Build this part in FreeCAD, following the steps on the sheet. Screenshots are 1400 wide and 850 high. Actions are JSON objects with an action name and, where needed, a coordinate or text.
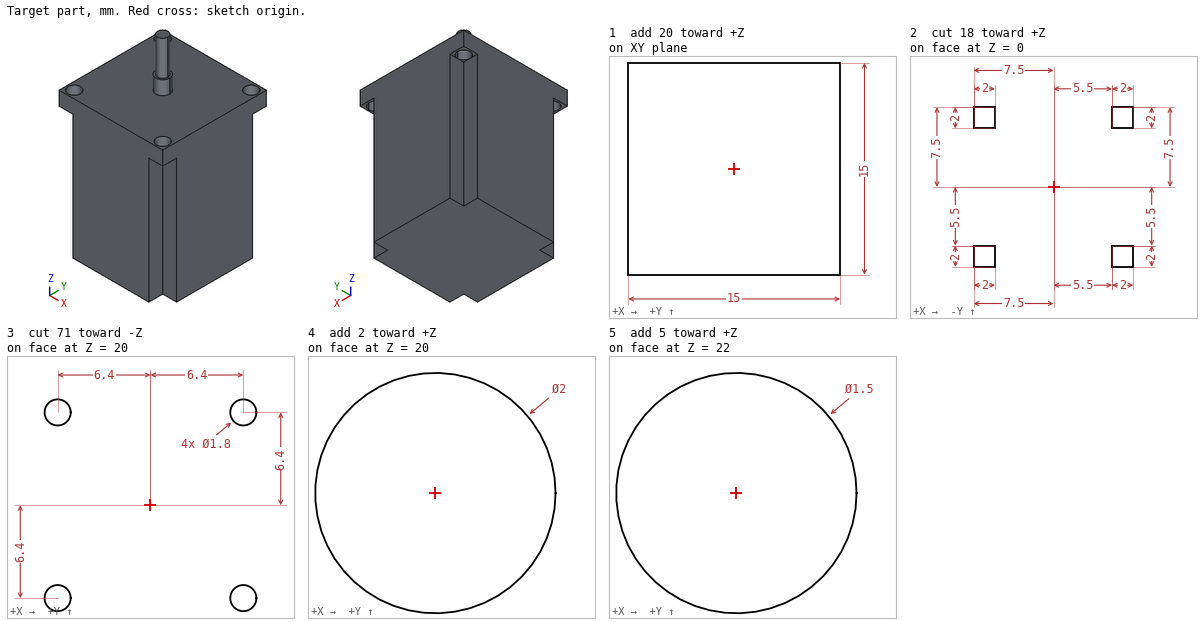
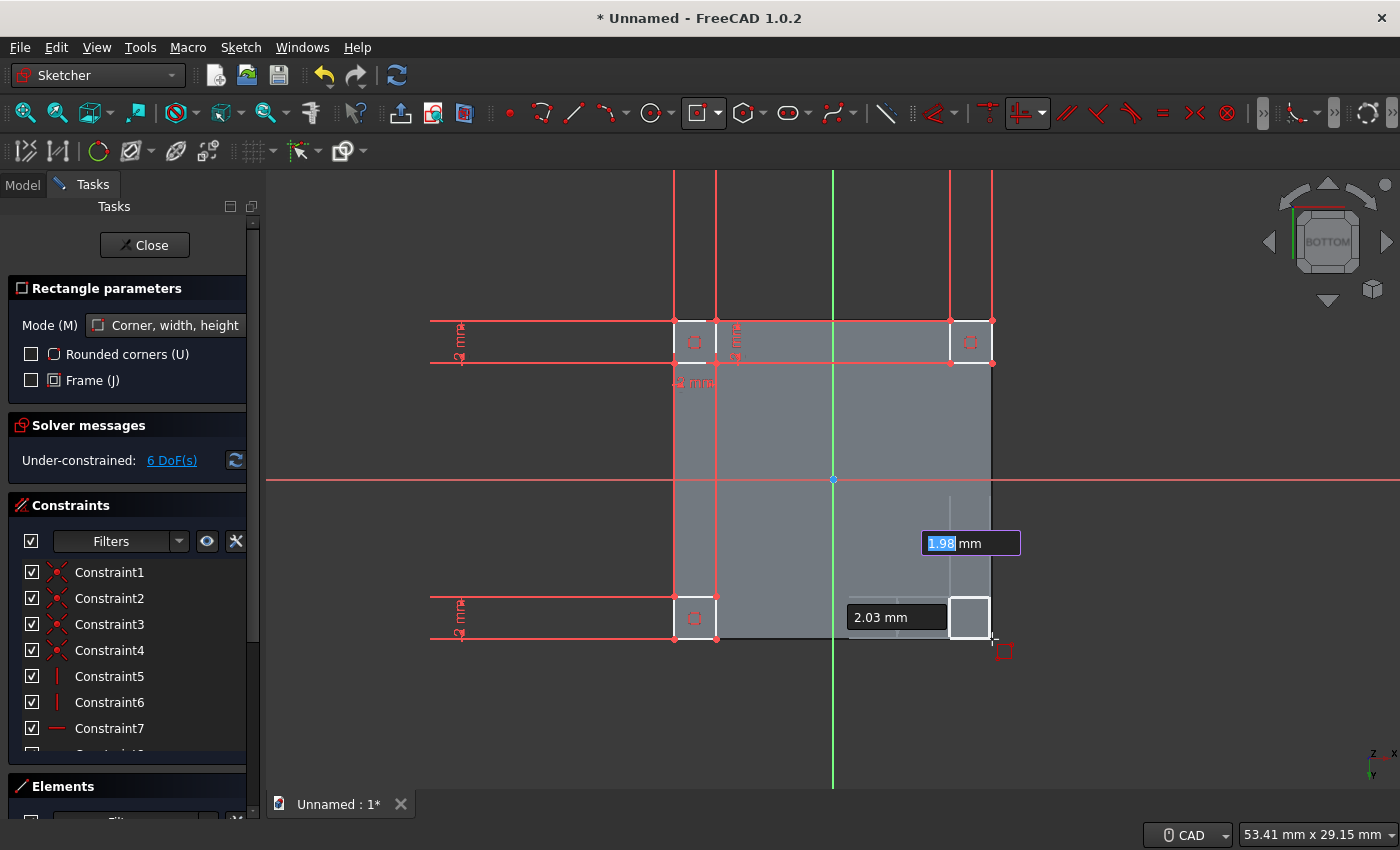
{"action": "type", "text": "2"}
{"action": "key", "text": "Tab"}
{"action": "type", "text": "2"}
{"action": "key", "text": "Return"}
{"action": "key", "text": "Escape"}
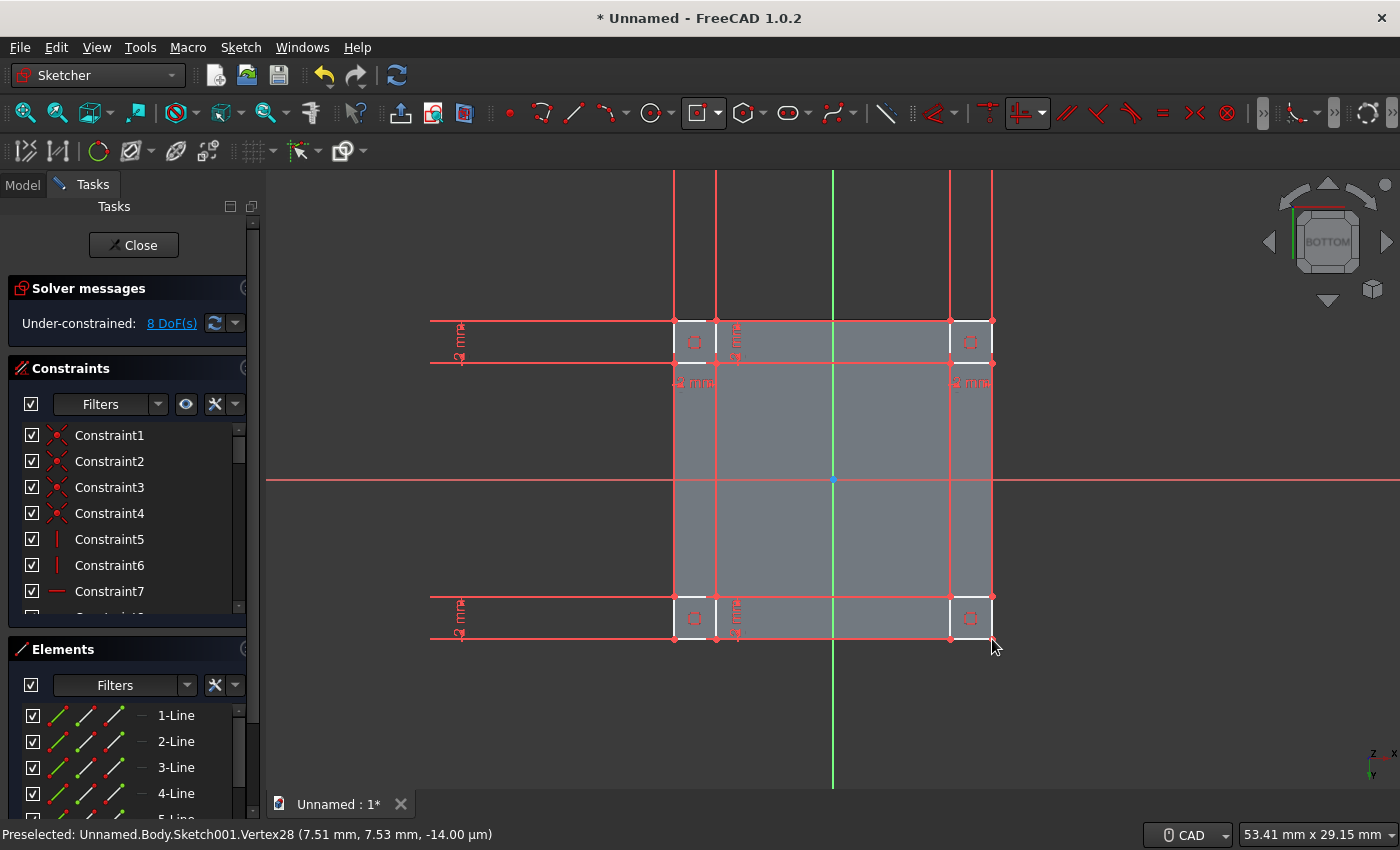
{"action": "left_click", "coordinate": [934, 114]}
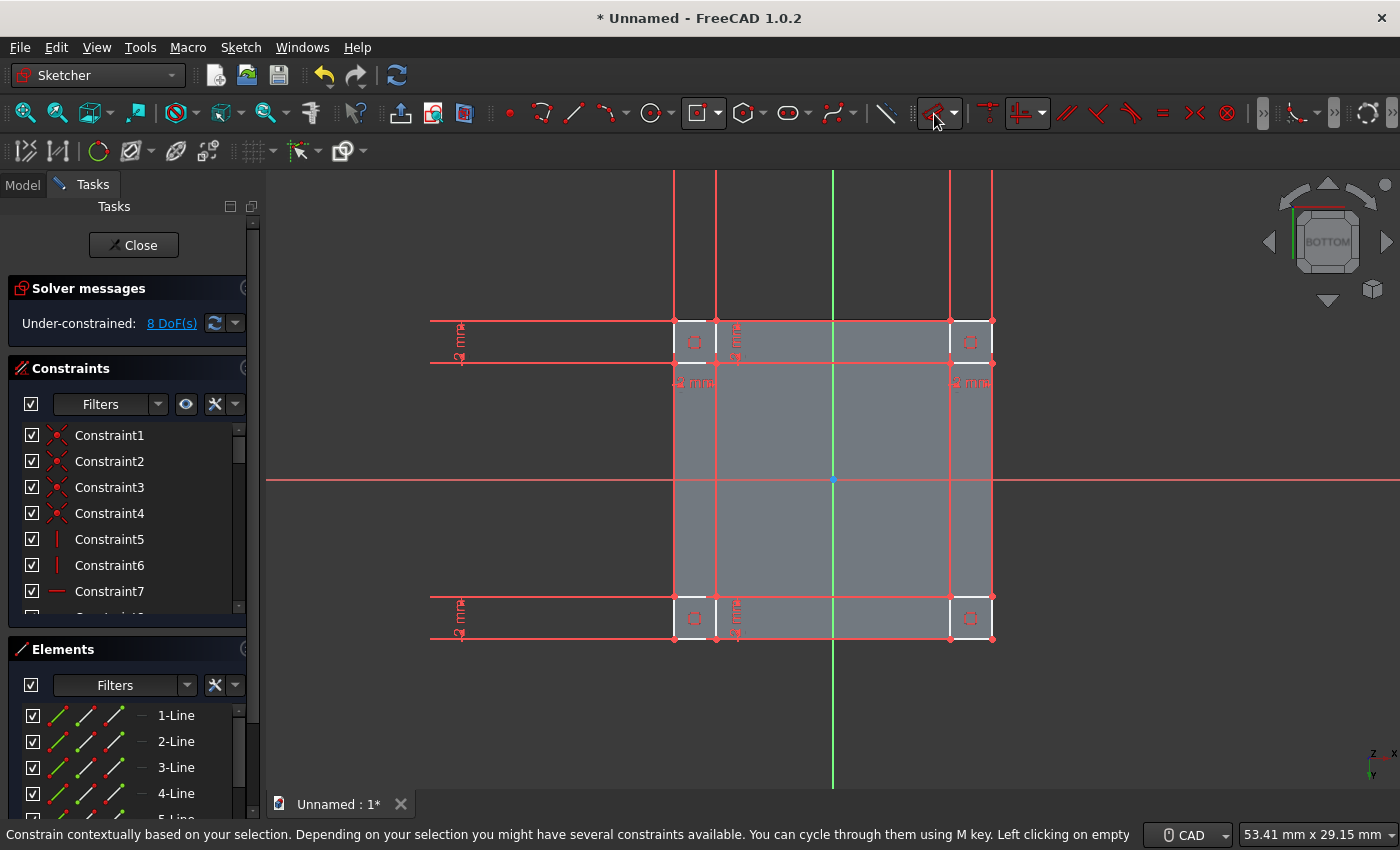
{"action": "left_click", "coordinate": [674, 597]}
{"action": "left_click", "coordinate": [754, 631]}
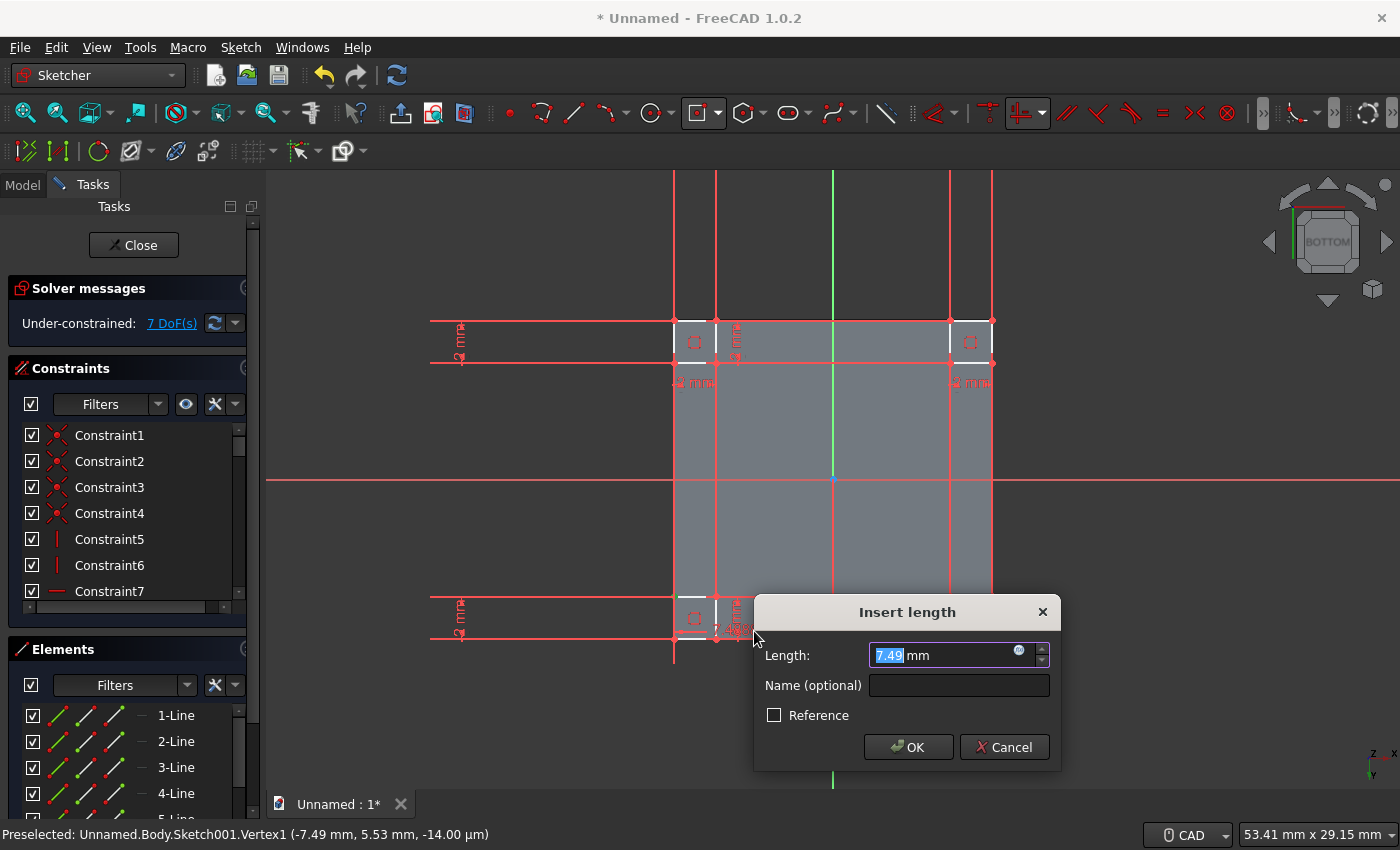
{"action": "type", "text": "7.5"}
{"action": "key", "text": "Return"}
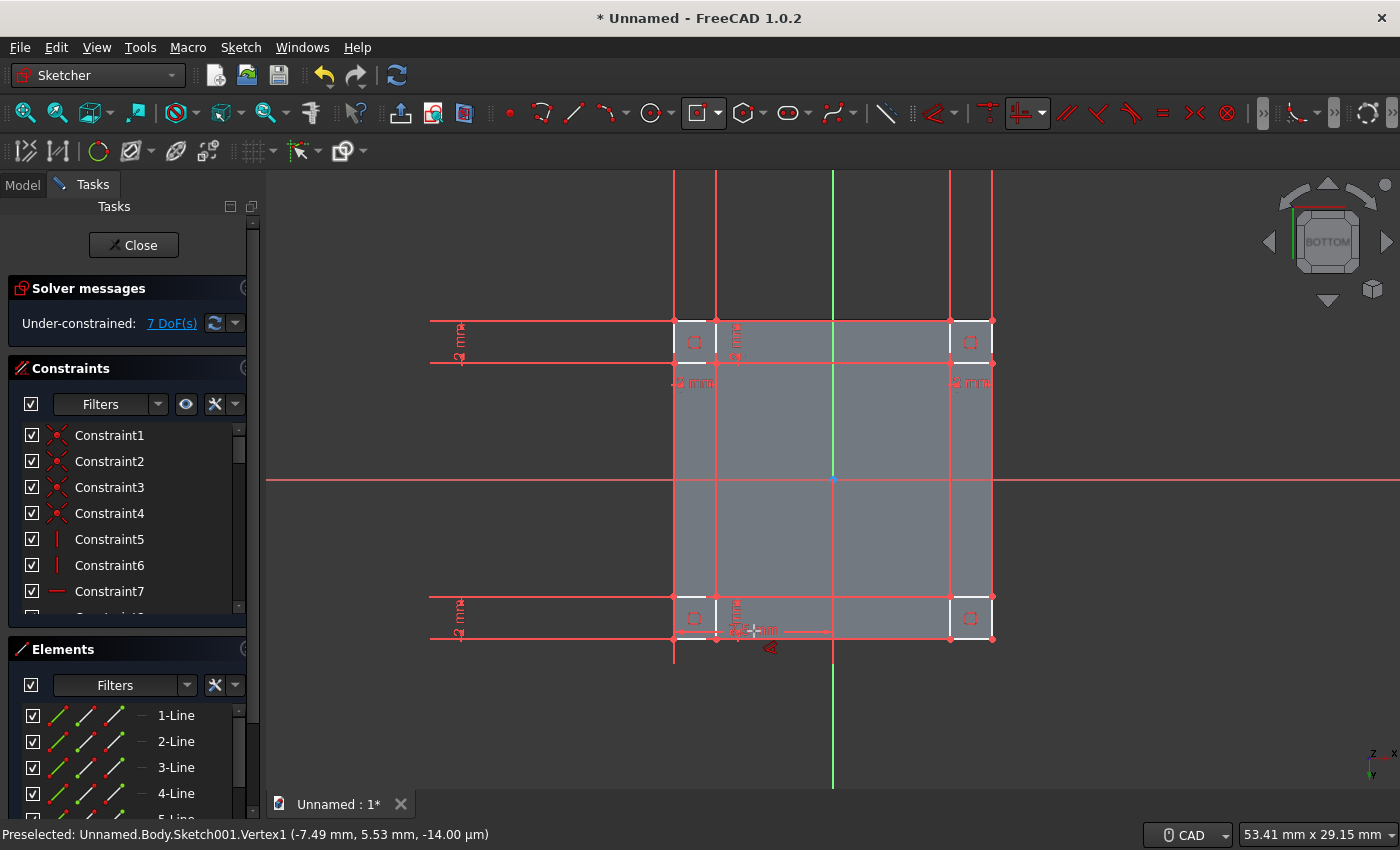
{"action": "left_click", "coordinate": [674, 597]}
{"action": "left_click", "coordinate": [640, 538]}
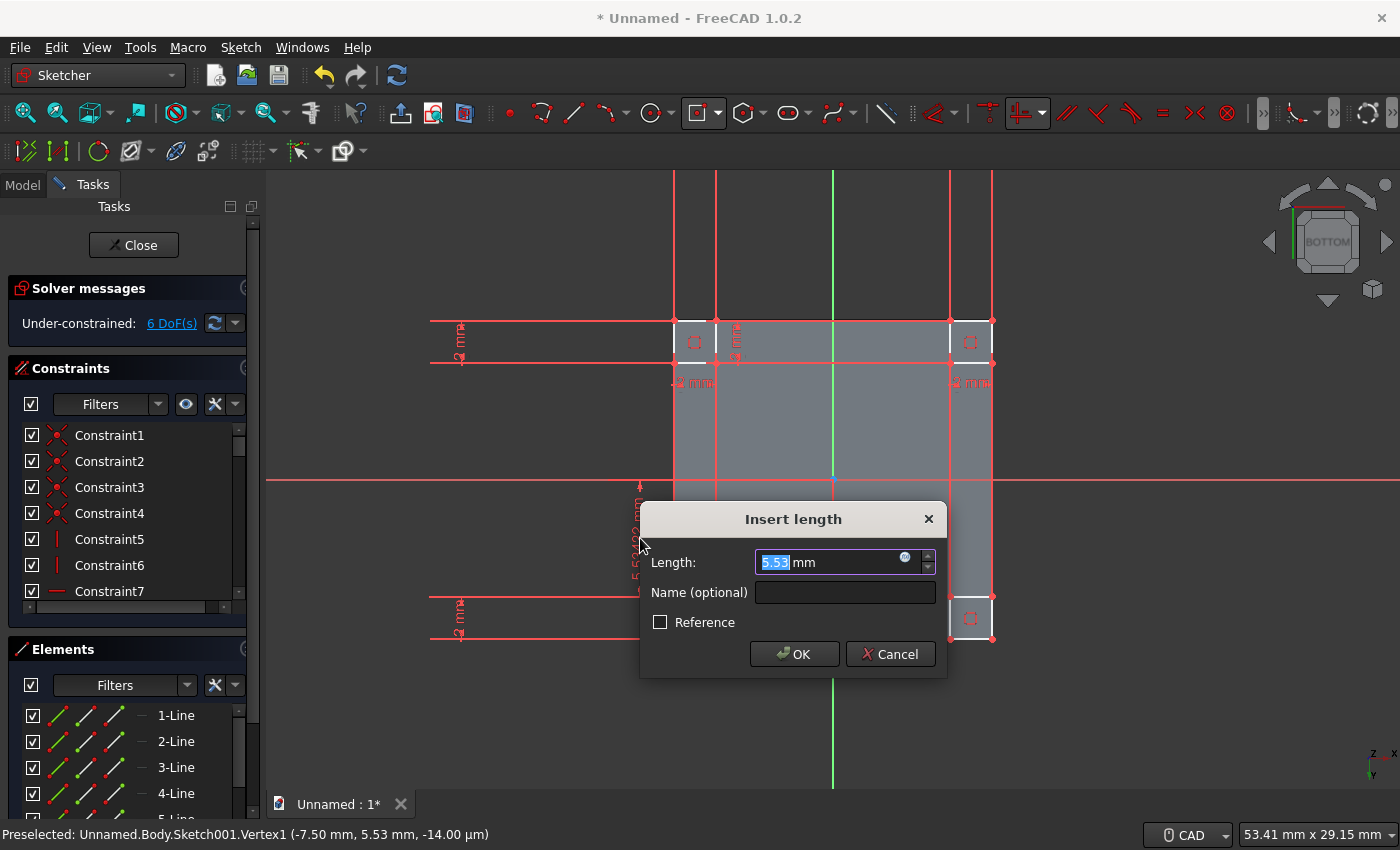
{"action": "type", "text": "5.5"}
{"action": "key", "text": "Return"}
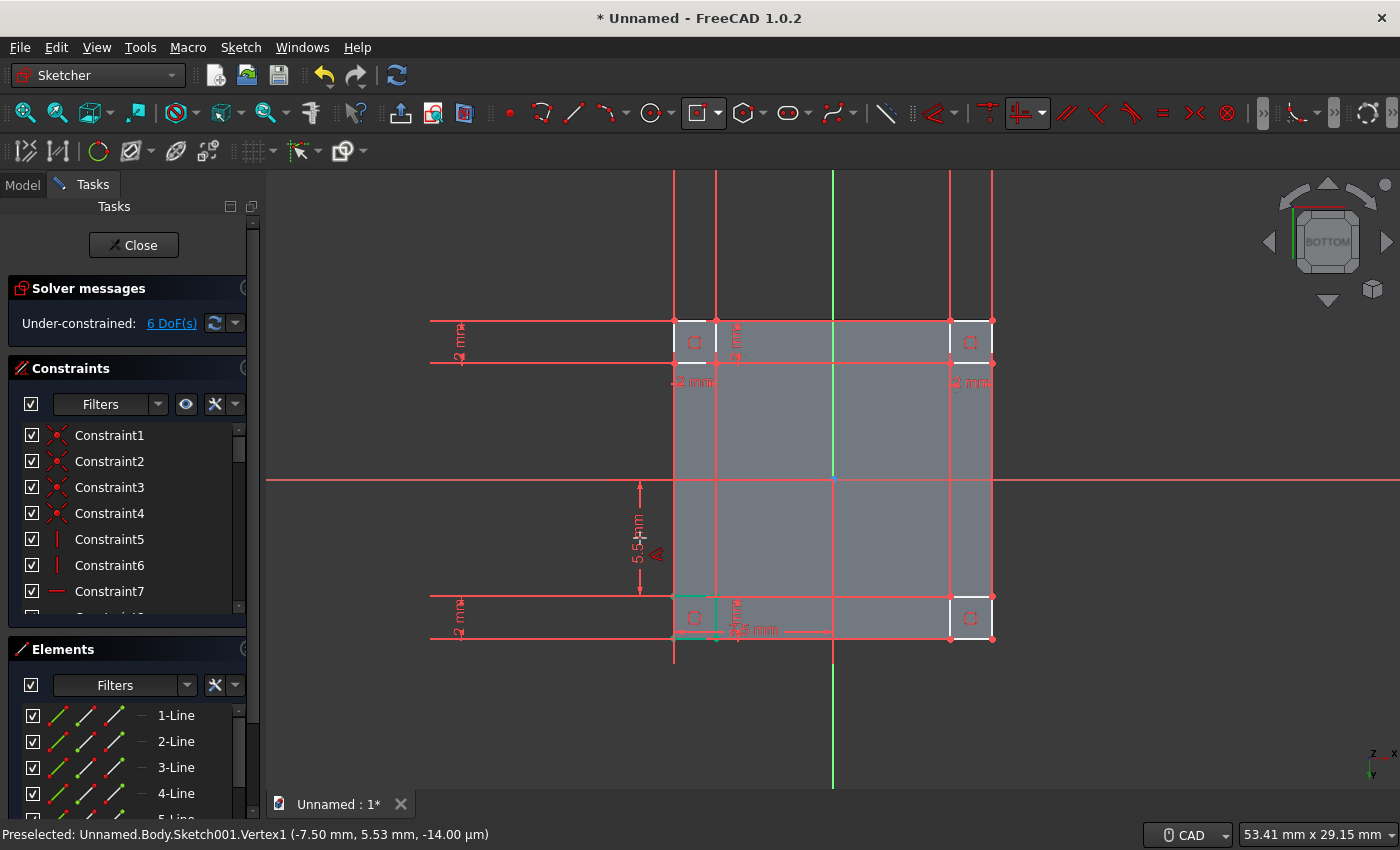
{"action": "left_click", "coordinate": [674, 321]}
{"action": "left_click", "coordinate": [754, 287]}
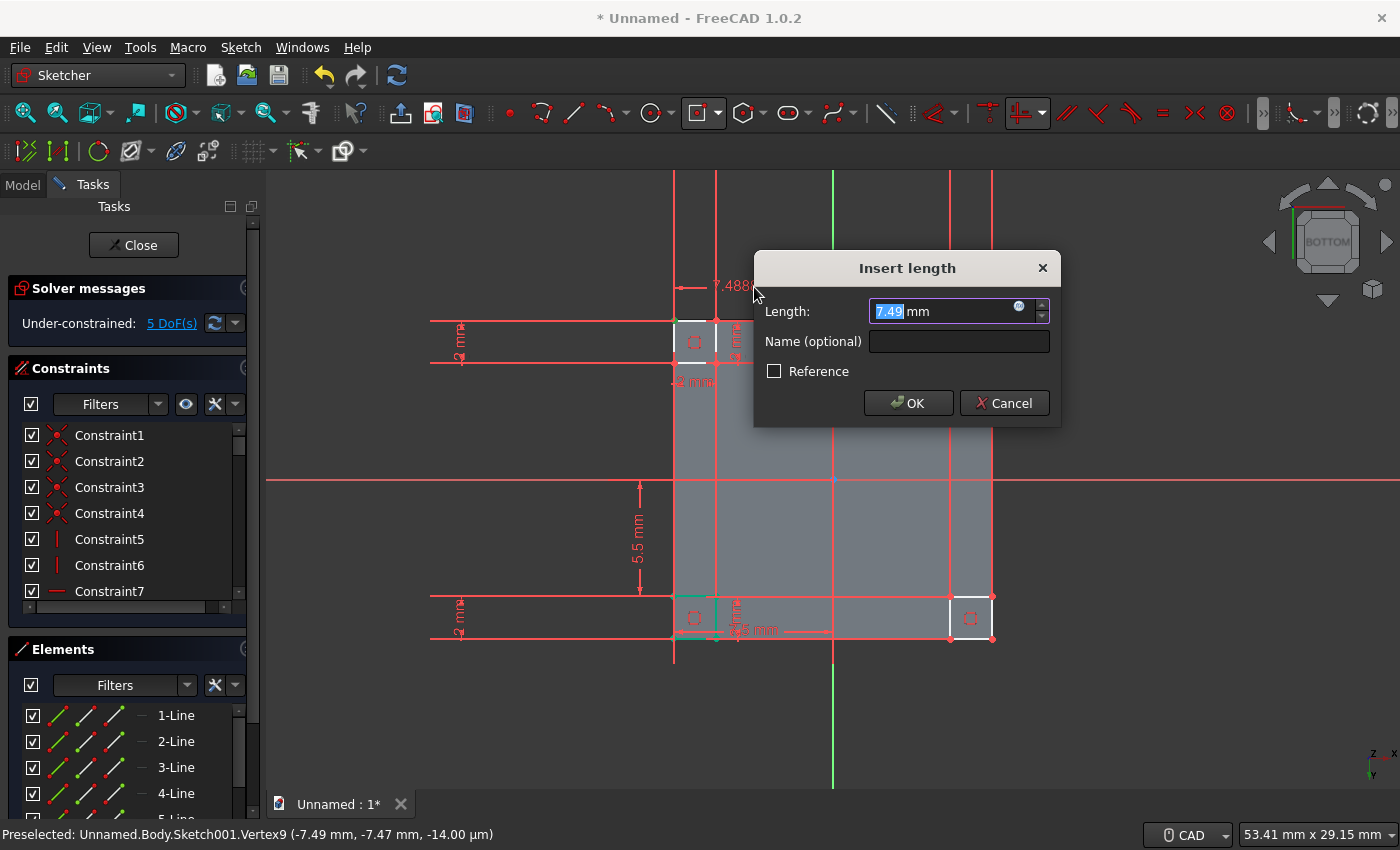
{"action": "type", "text": "7.5"}
{"action": "key", "text": "Return"}